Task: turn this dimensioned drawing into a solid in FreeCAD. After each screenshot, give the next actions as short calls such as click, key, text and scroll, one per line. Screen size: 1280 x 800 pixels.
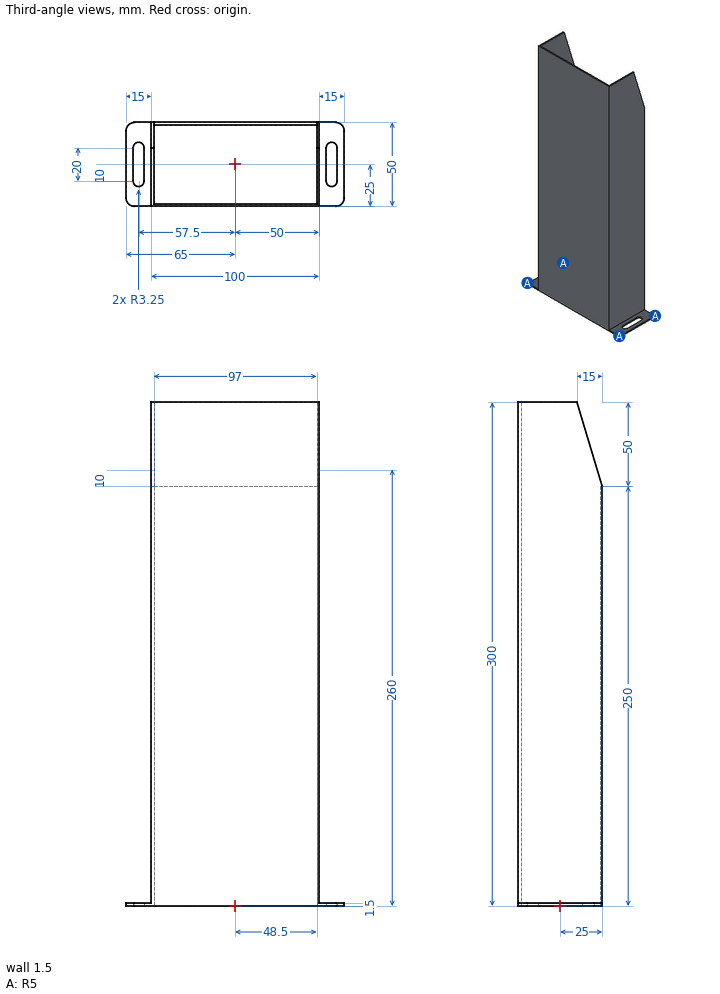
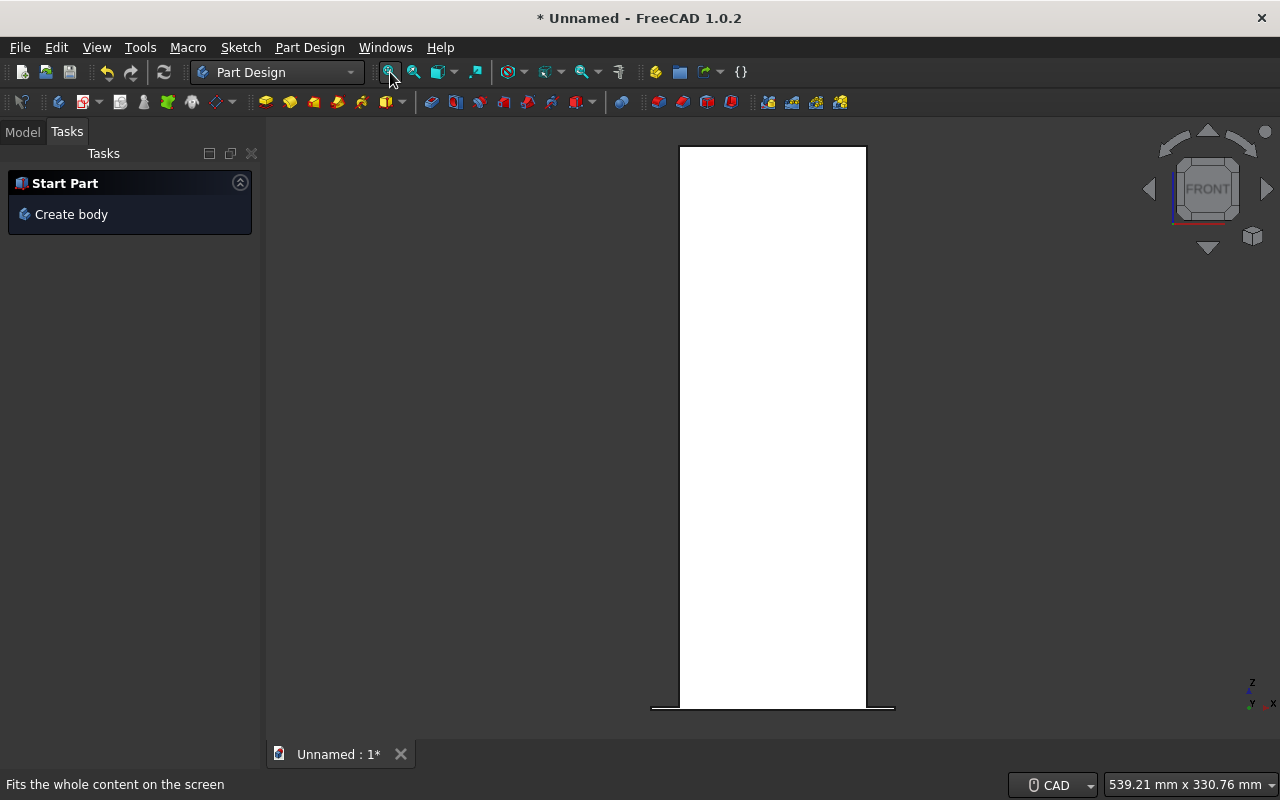
scroll(895, 708, up, 14)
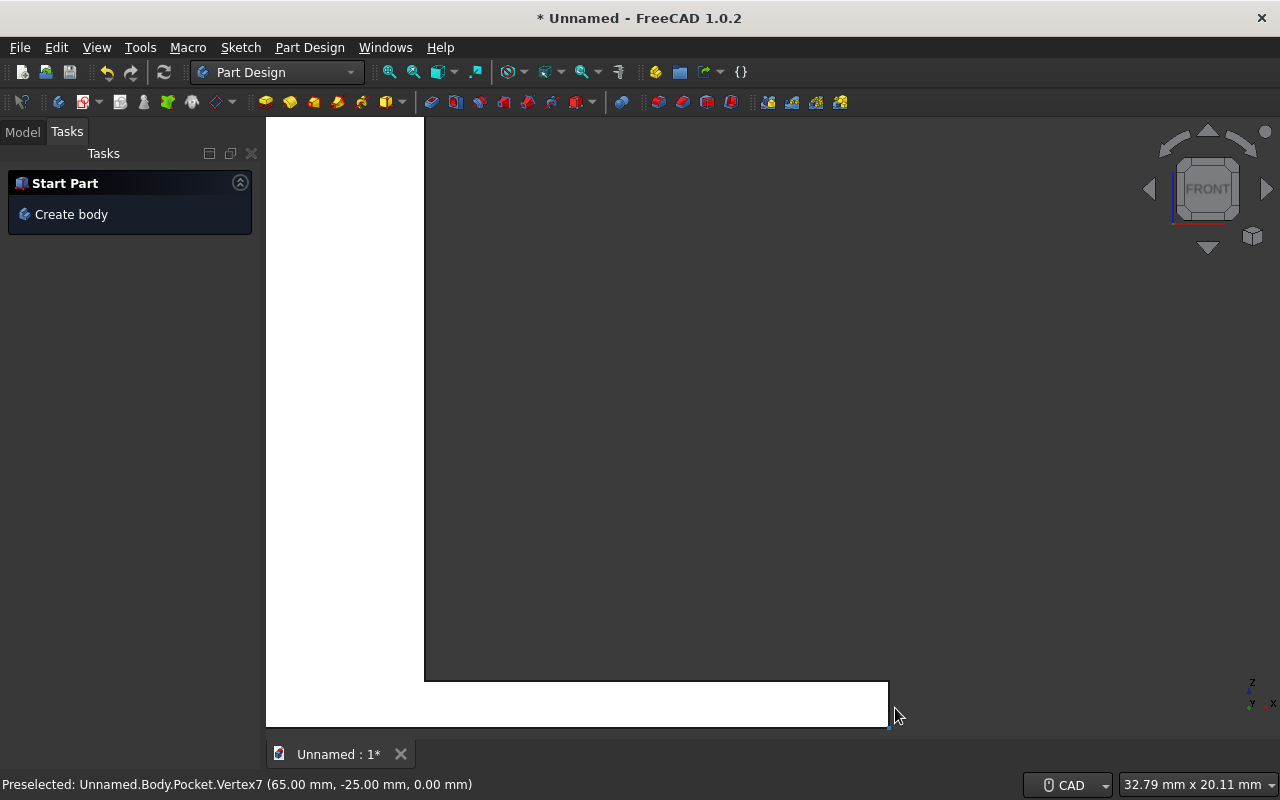
click(889, 703)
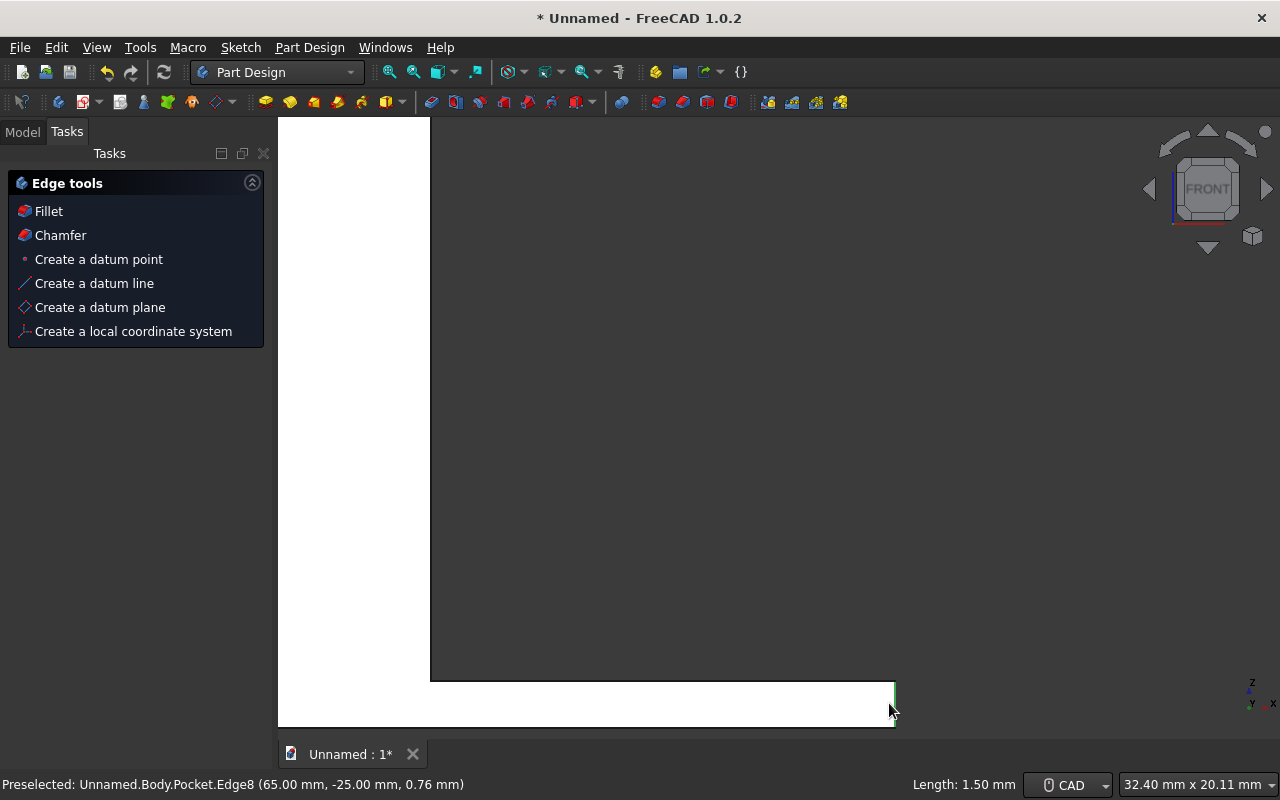
click(390, 72)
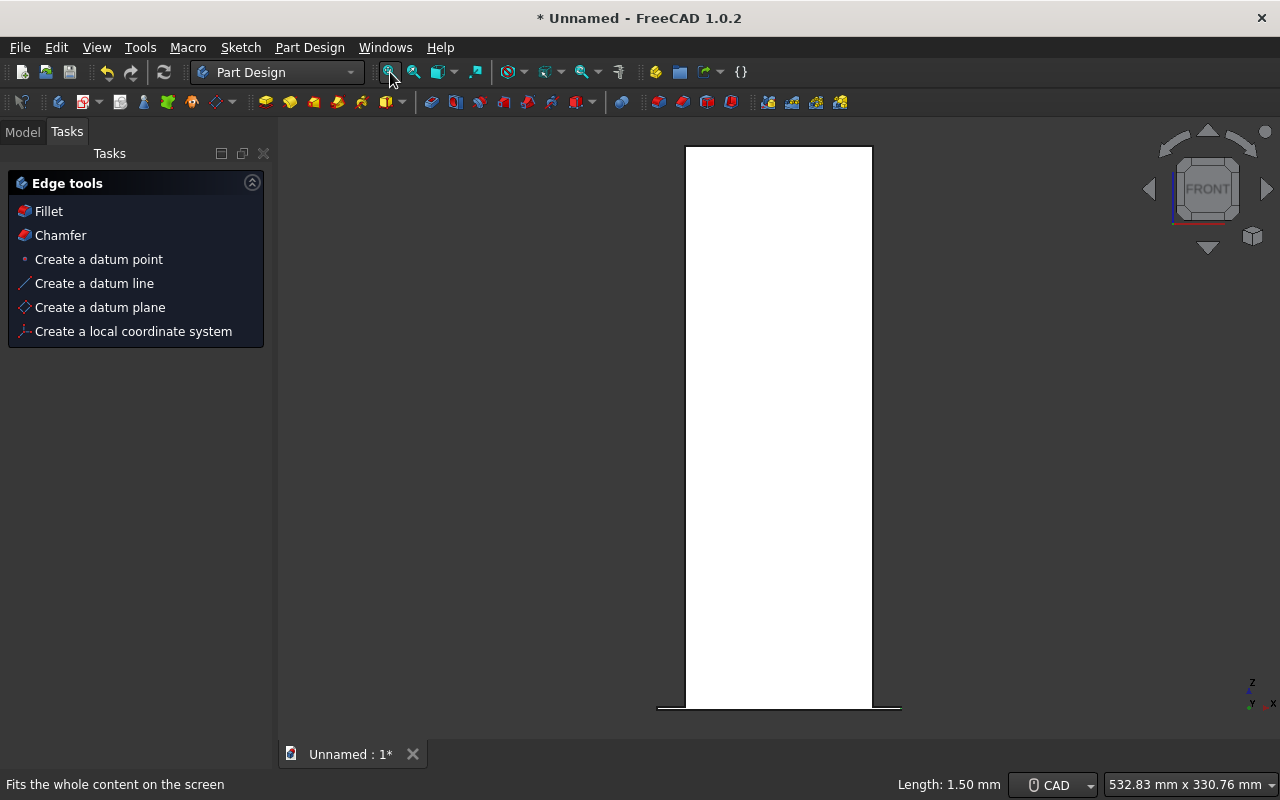
key(3)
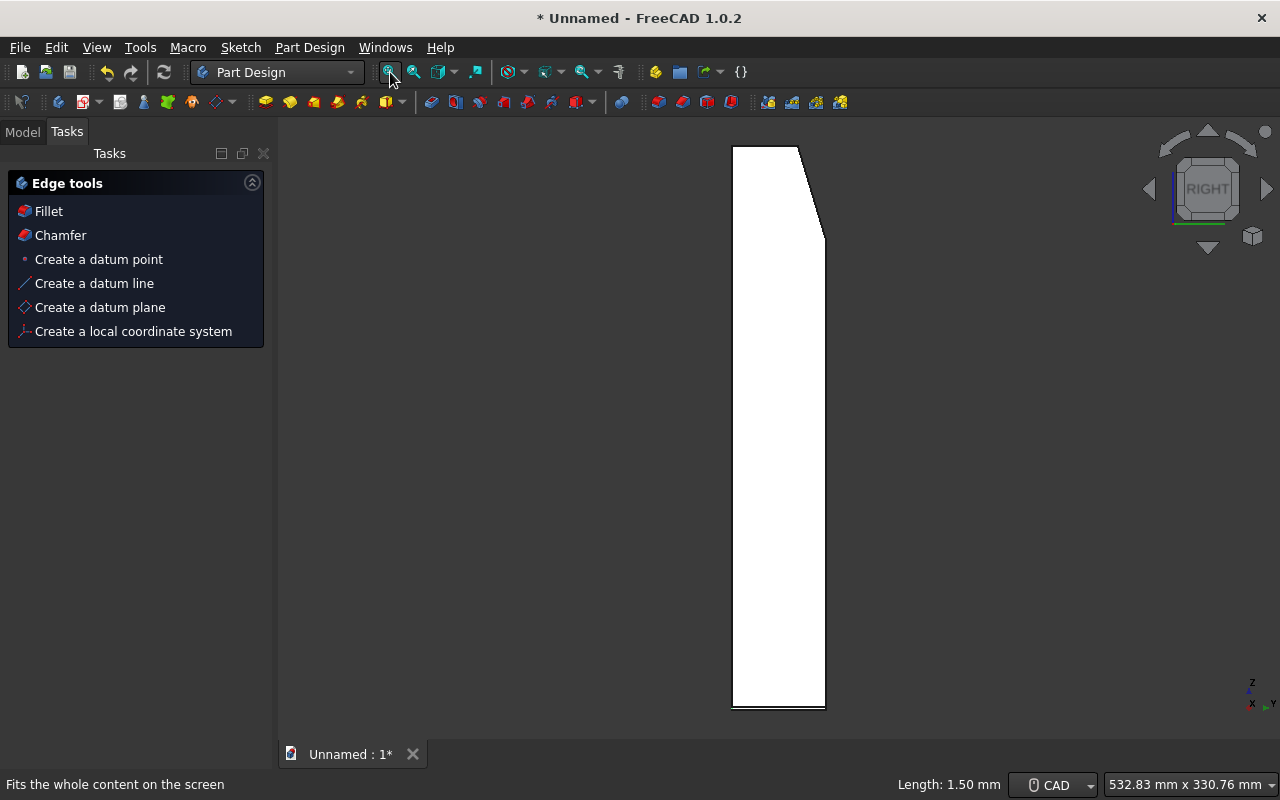
scroll(826, 708, up, 14)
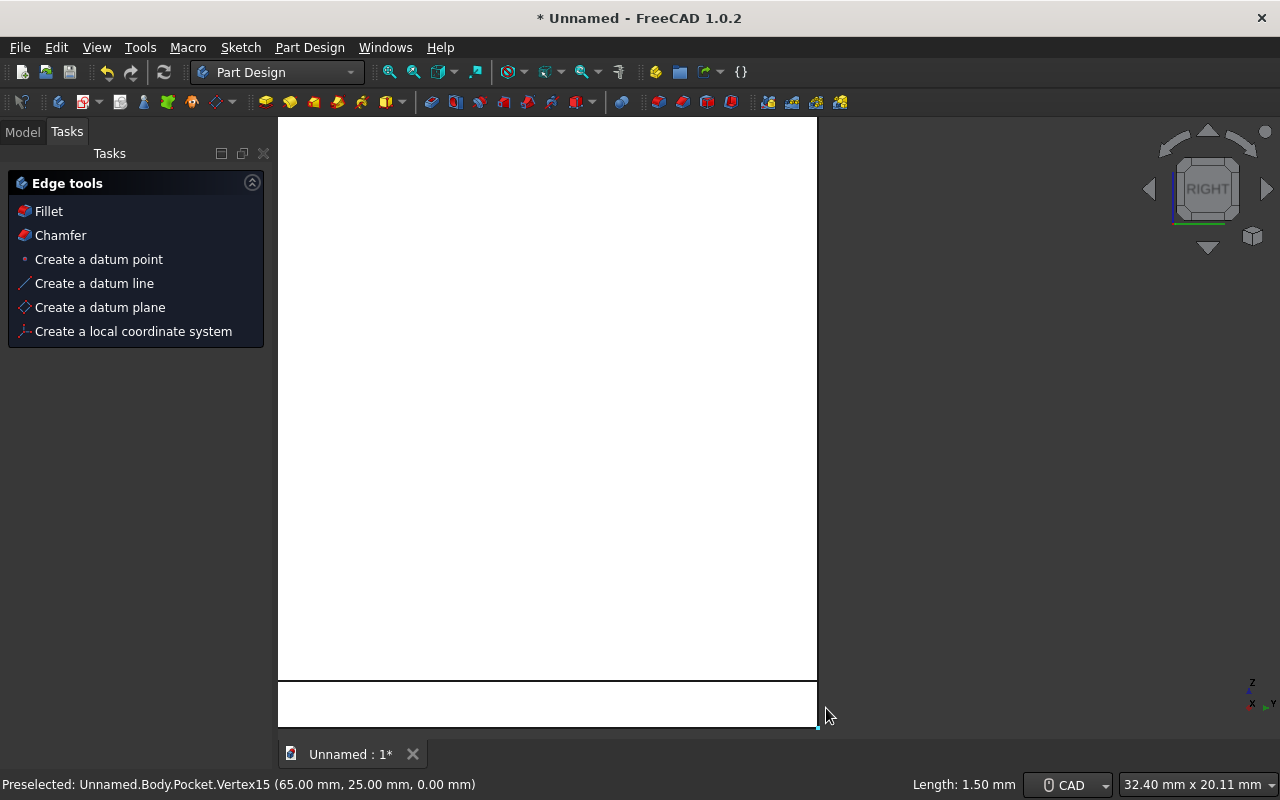
click(818, 703, ctrl)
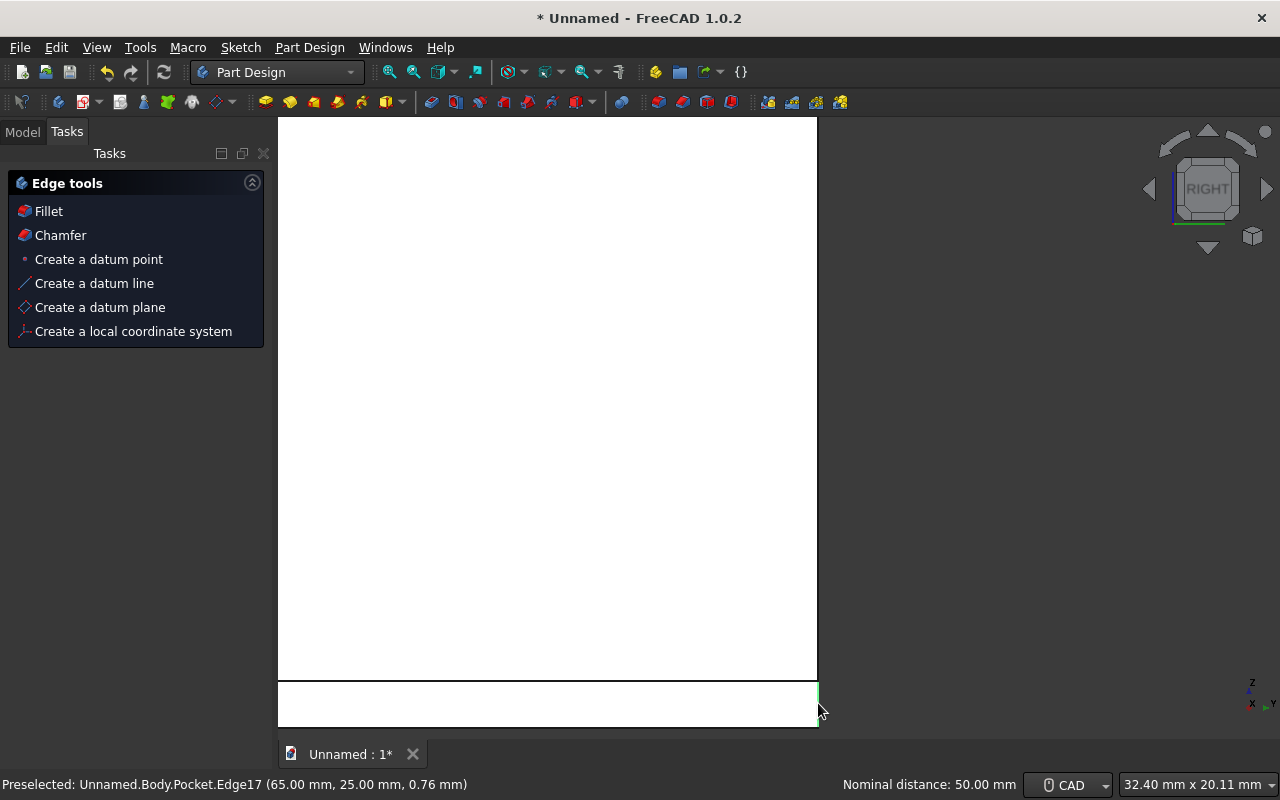
click(390, 72)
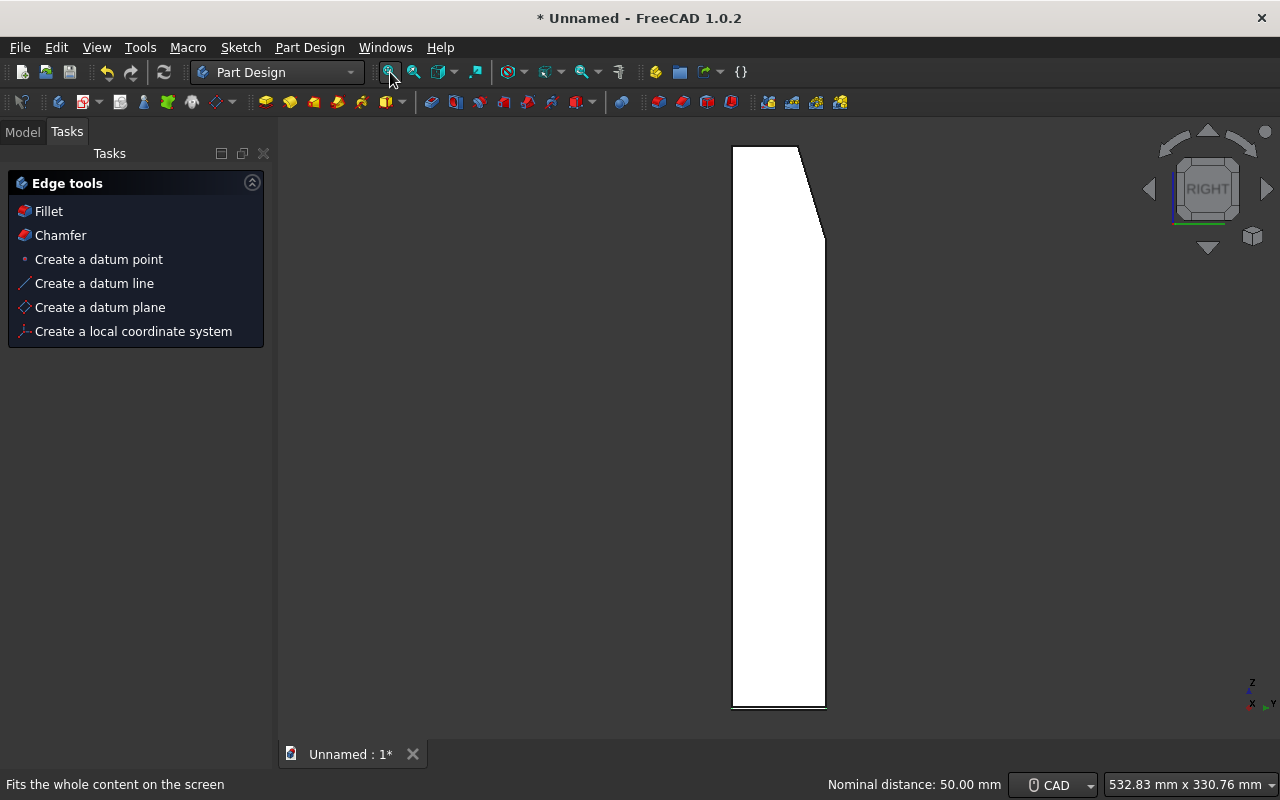
key(5)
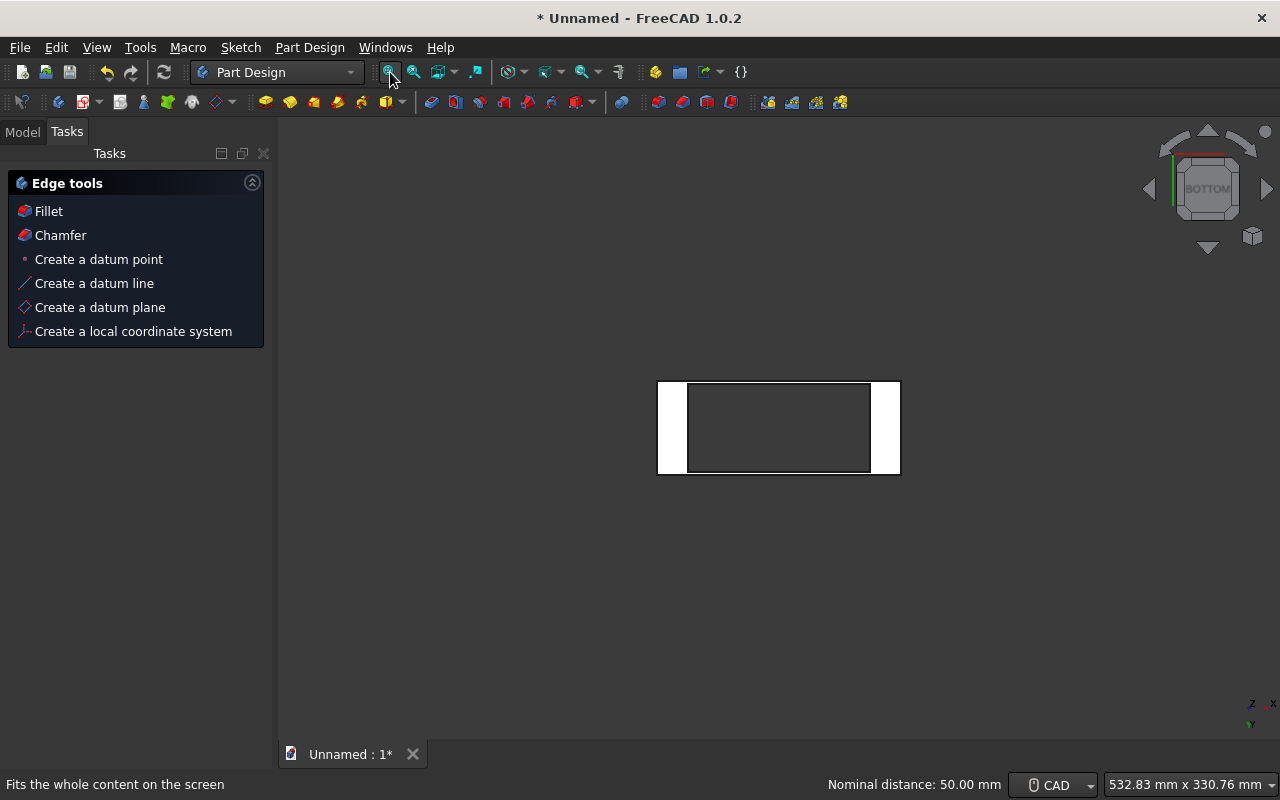
click(390, 72)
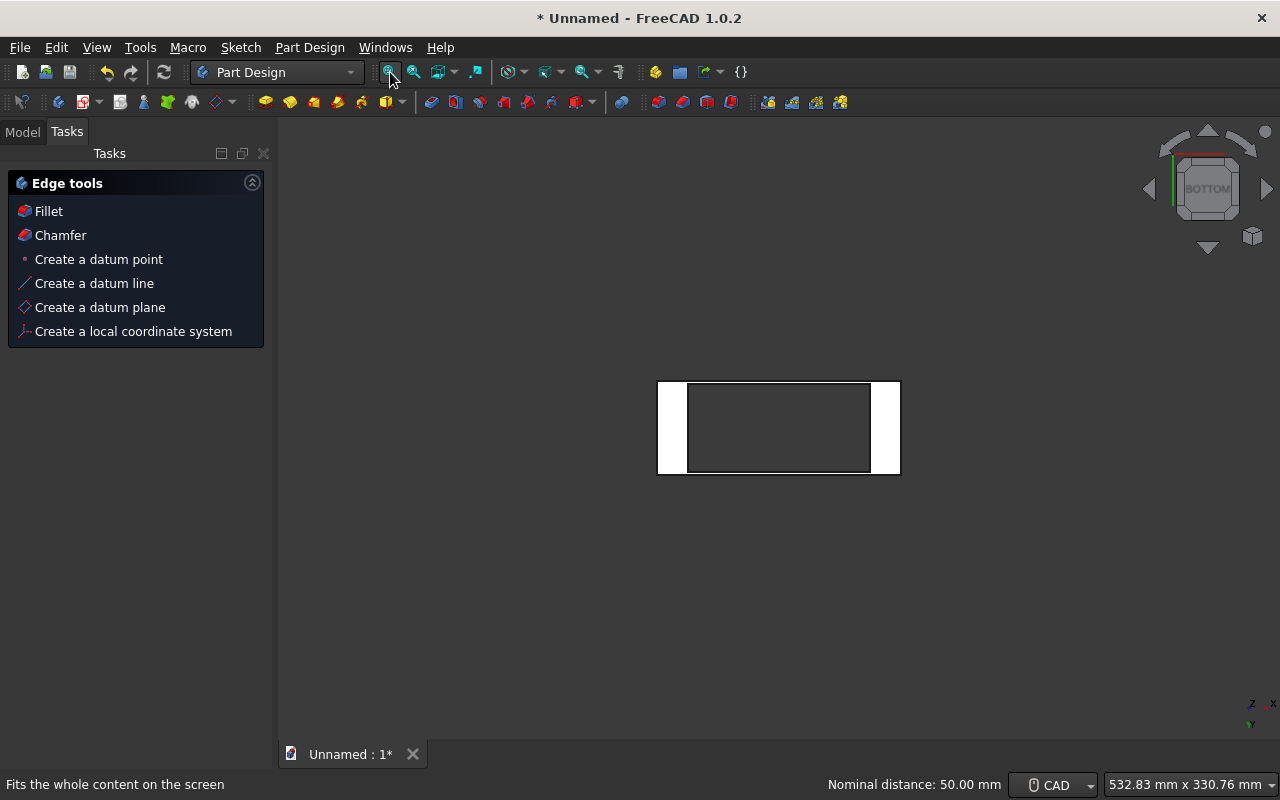
scroll(657, 474, up, 14)